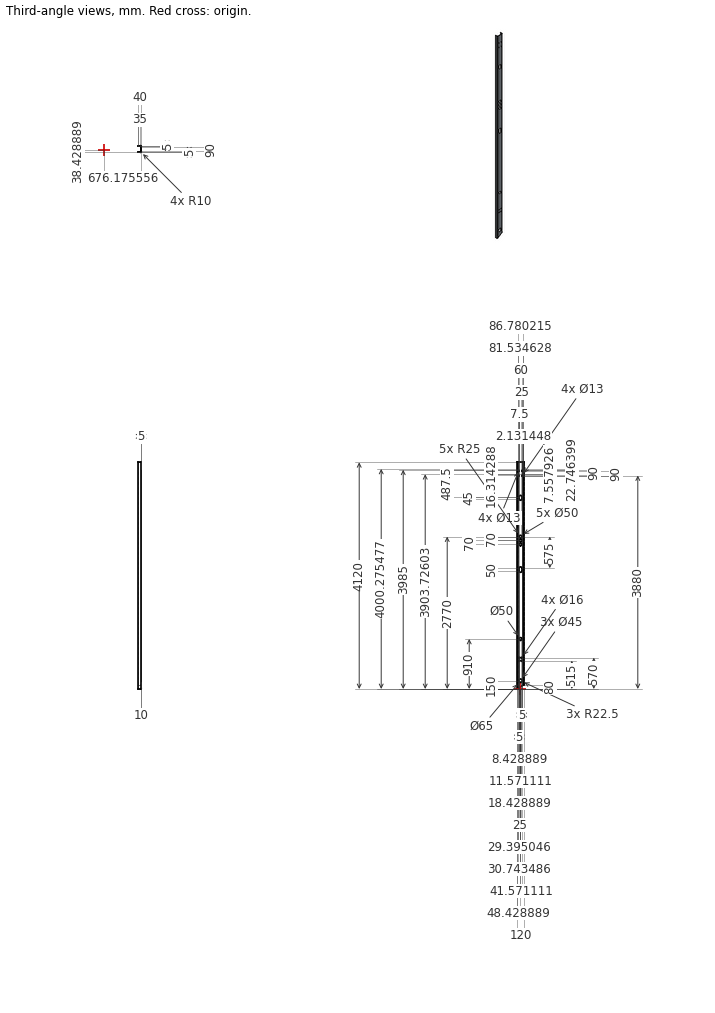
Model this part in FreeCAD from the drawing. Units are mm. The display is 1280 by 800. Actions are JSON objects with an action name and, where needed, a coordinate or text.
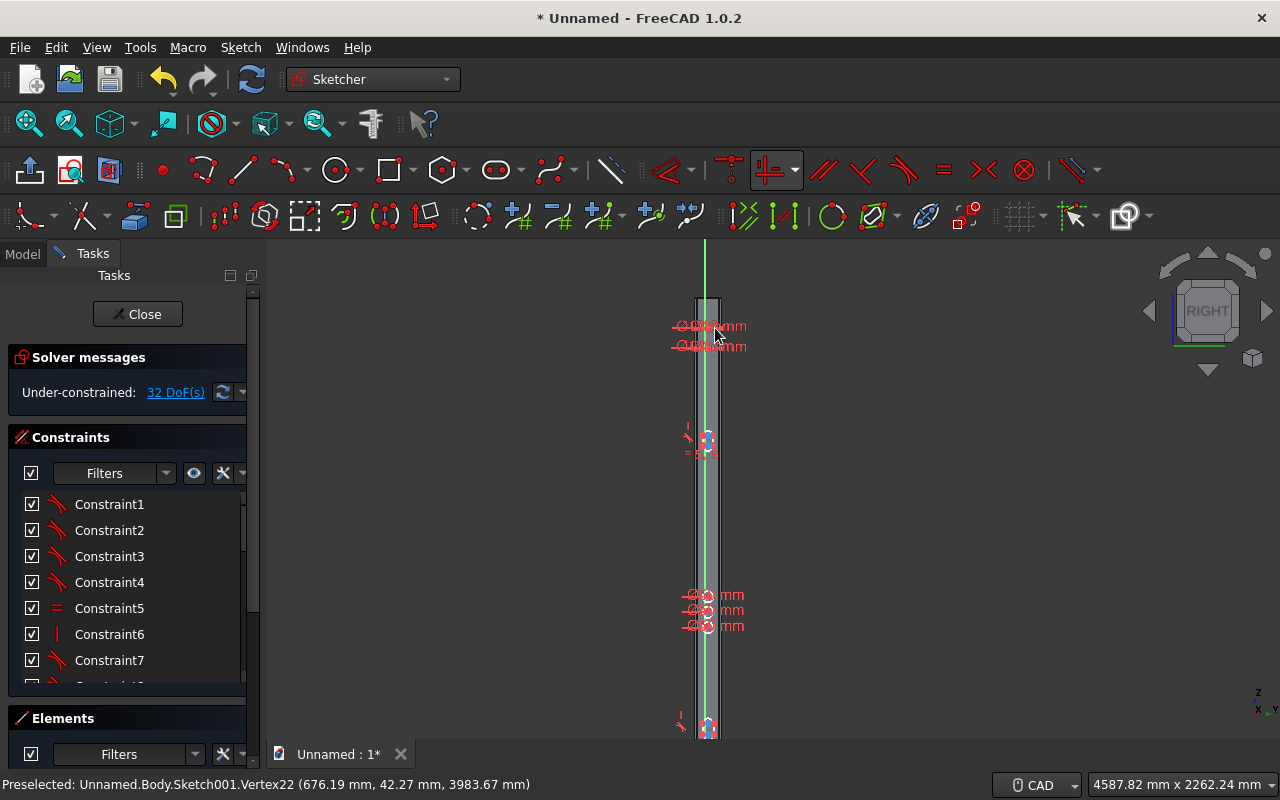
{"action": "key", "text": "h"}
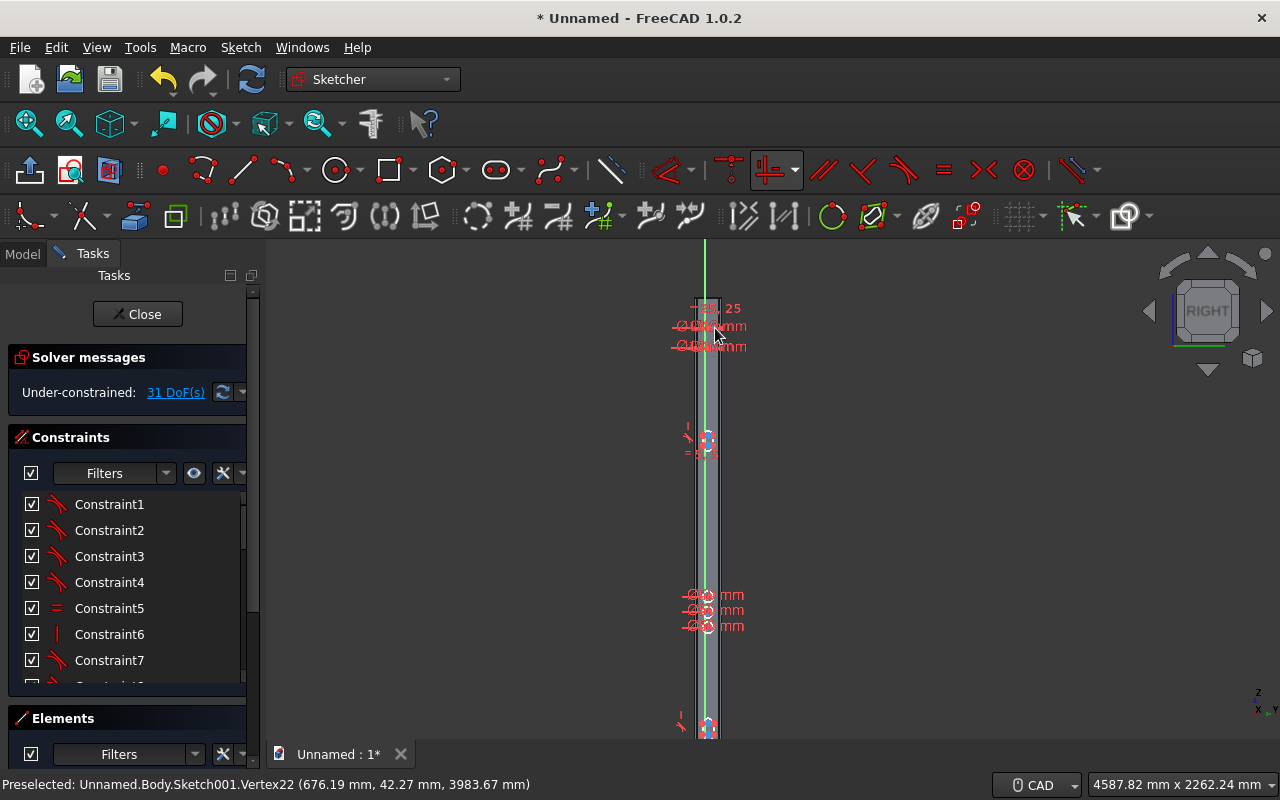
{"action": "left_click", "coordinate": [715, 328]}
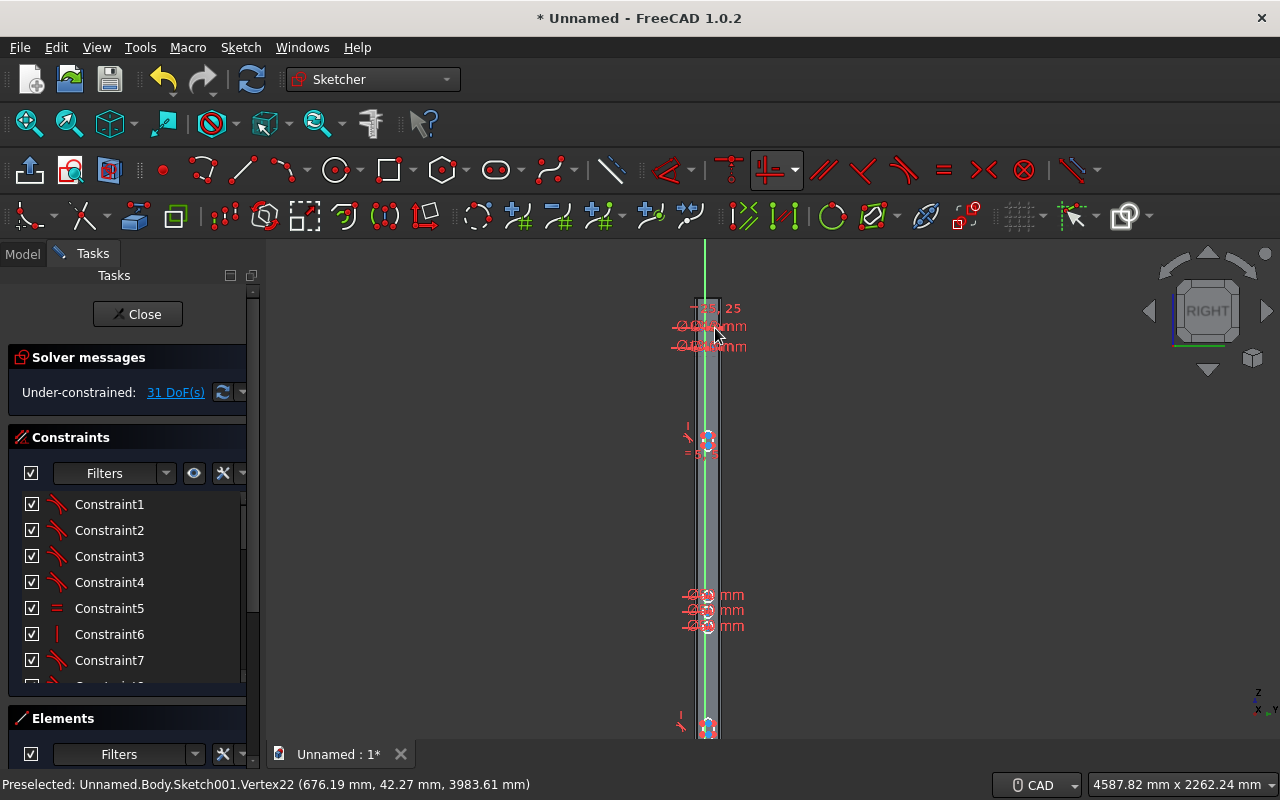
{"action": "left_click", "coordinate": [715, 349]}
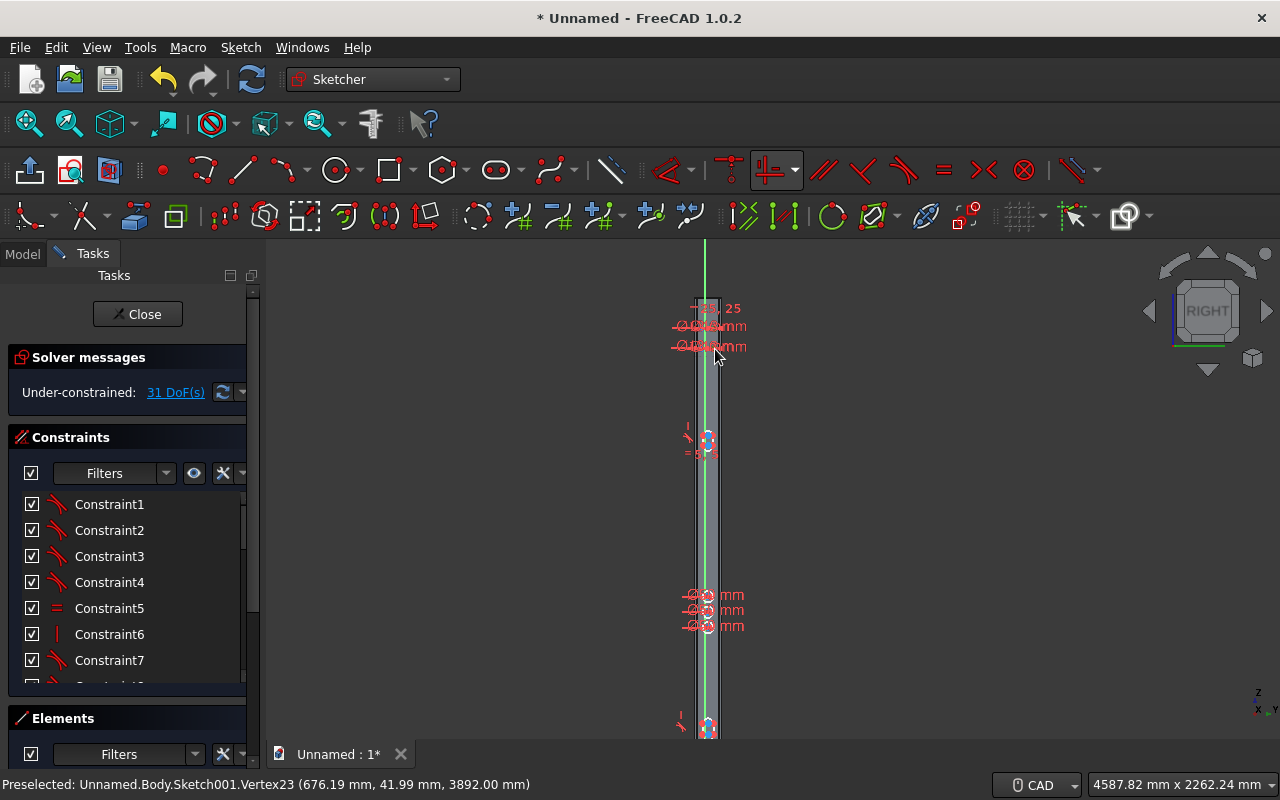
{"action": "left_click", "coordinate": [798, 170]}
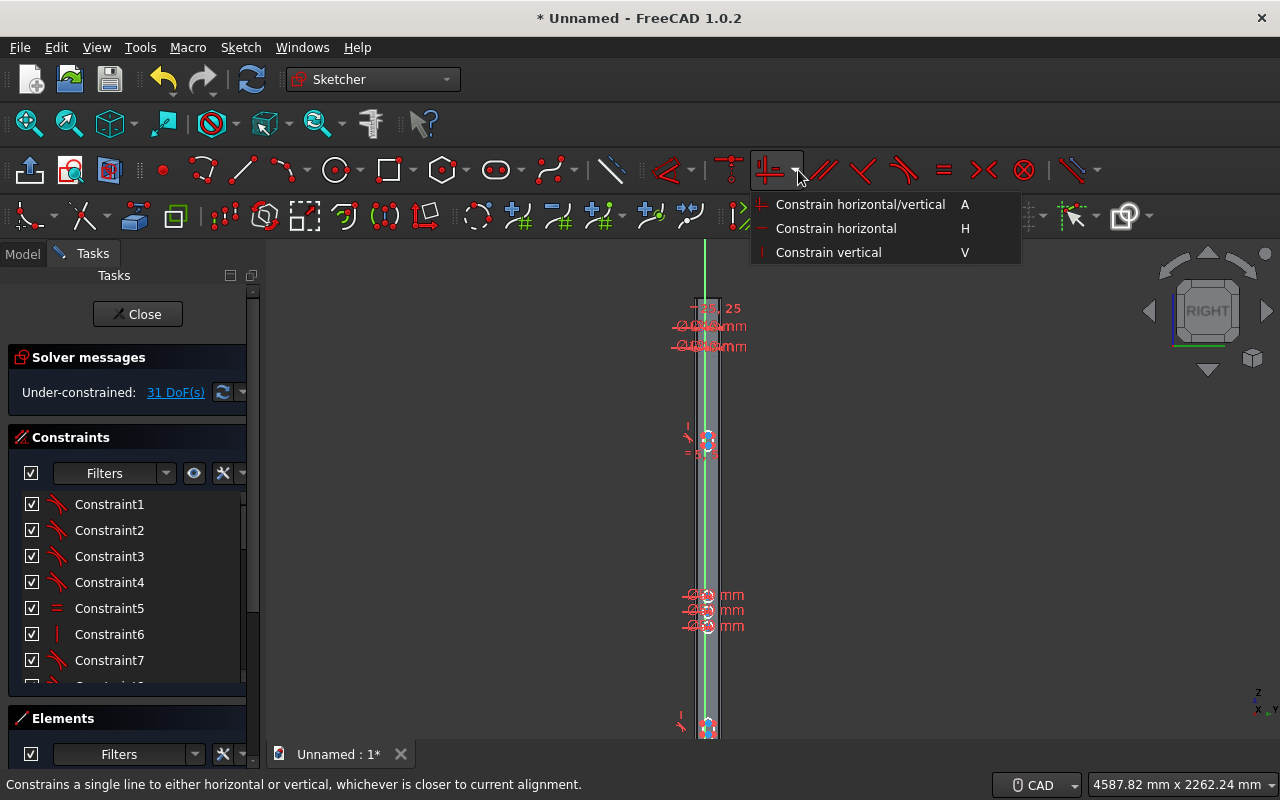
{"action": "left_click", "coordinate": [886, 252]}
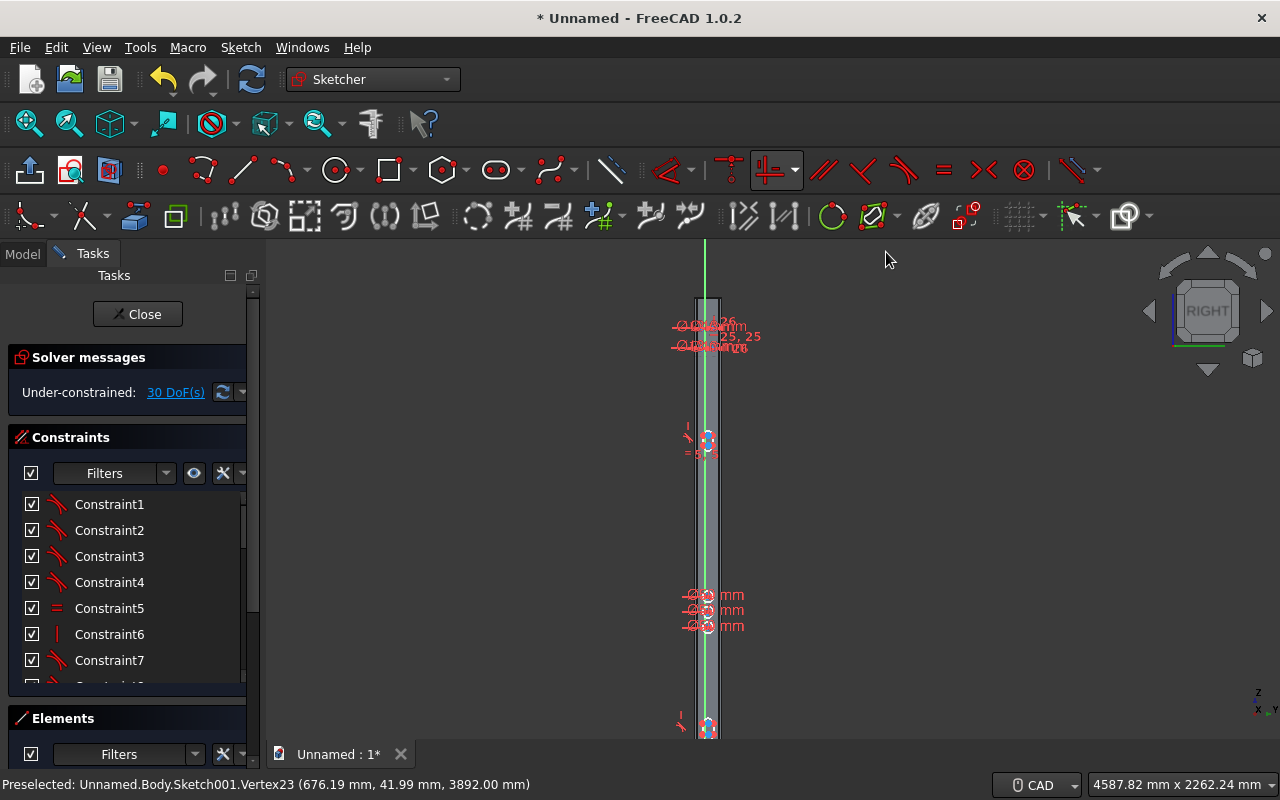
{"action": "left_click", "coordinate": [701, 328]}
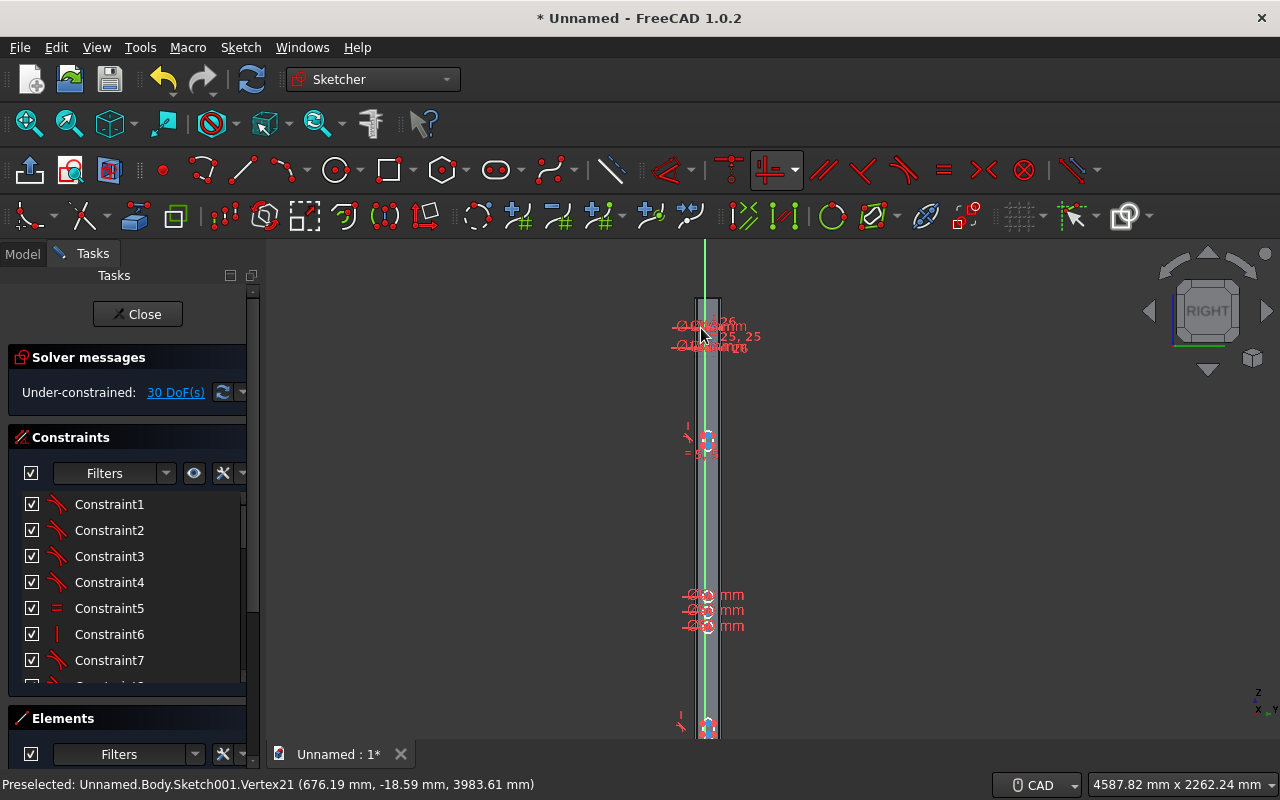
{"action": "left_click", "coordinate": [701, 348]}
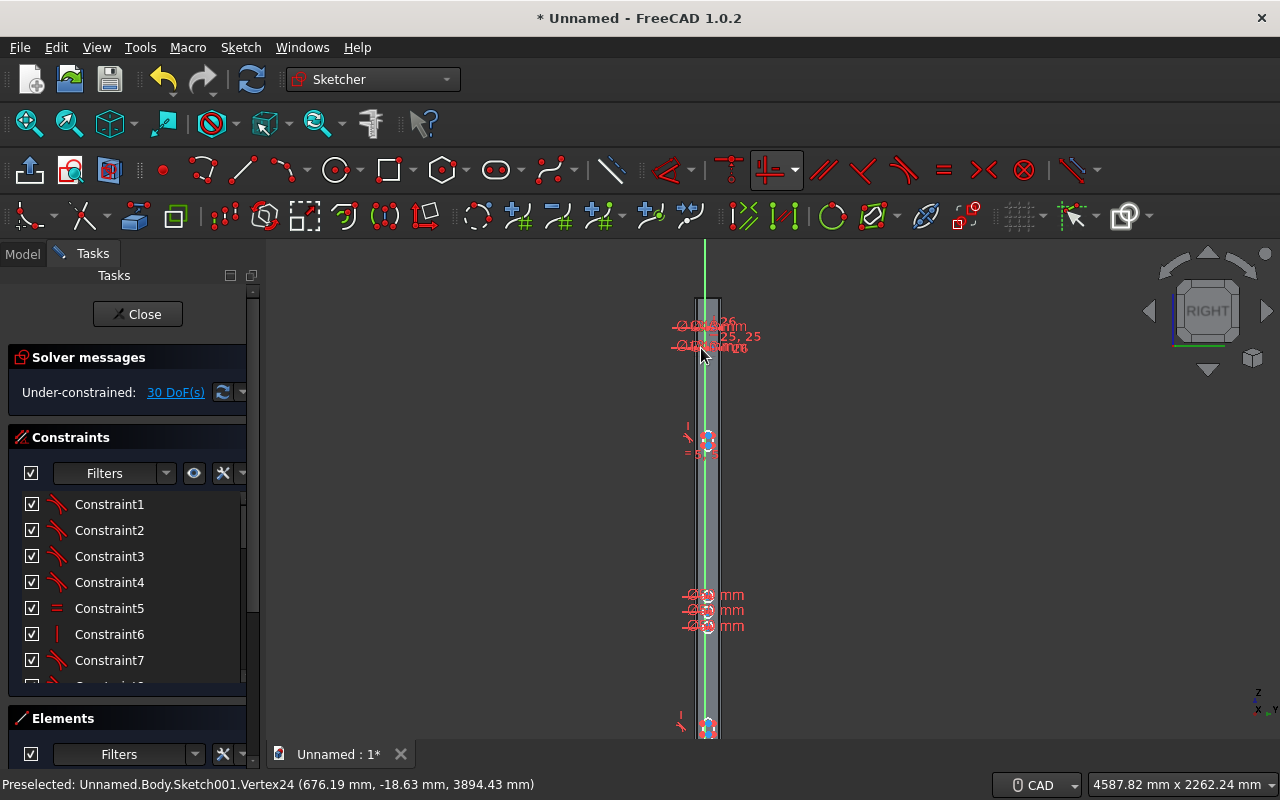
{"action": "key", "text": "v"}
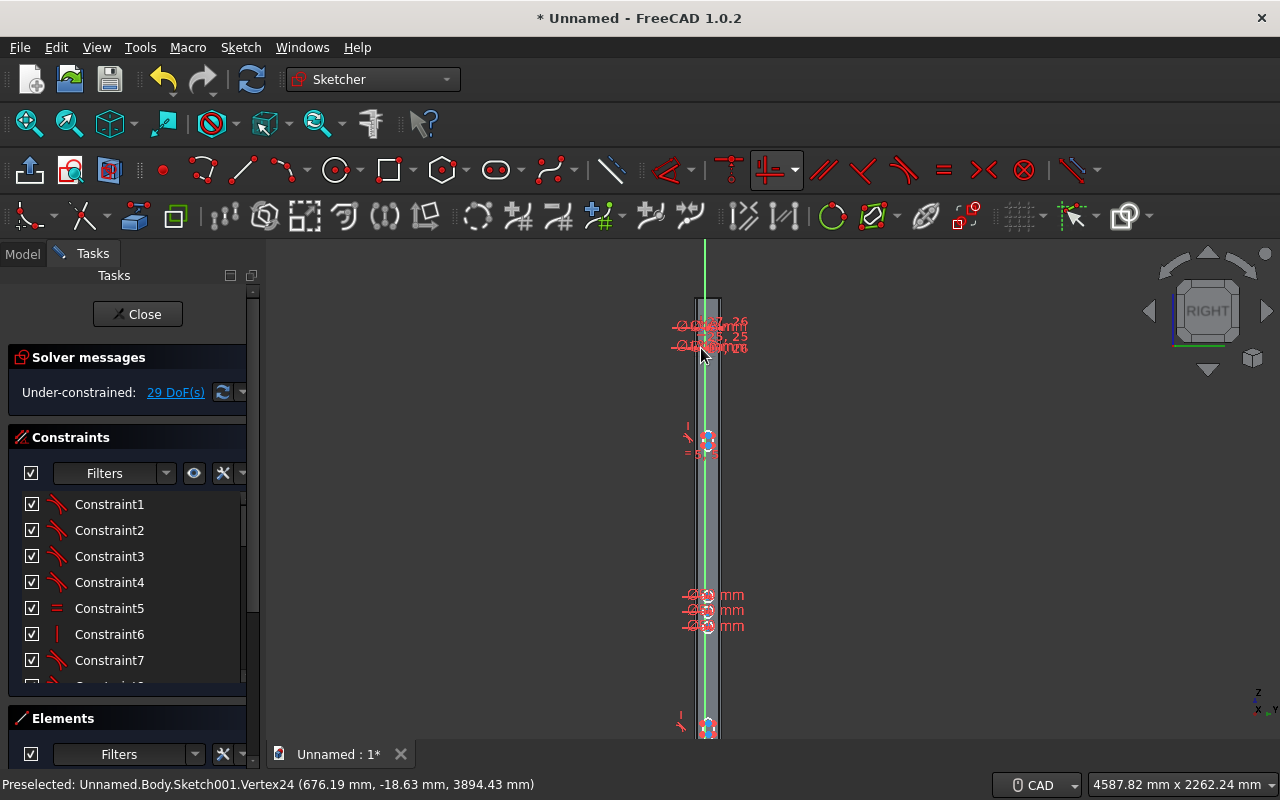
{"action": "scroll", "coordinate": [715, 349], "scroll_direction": "up", "scroll_amount": 4}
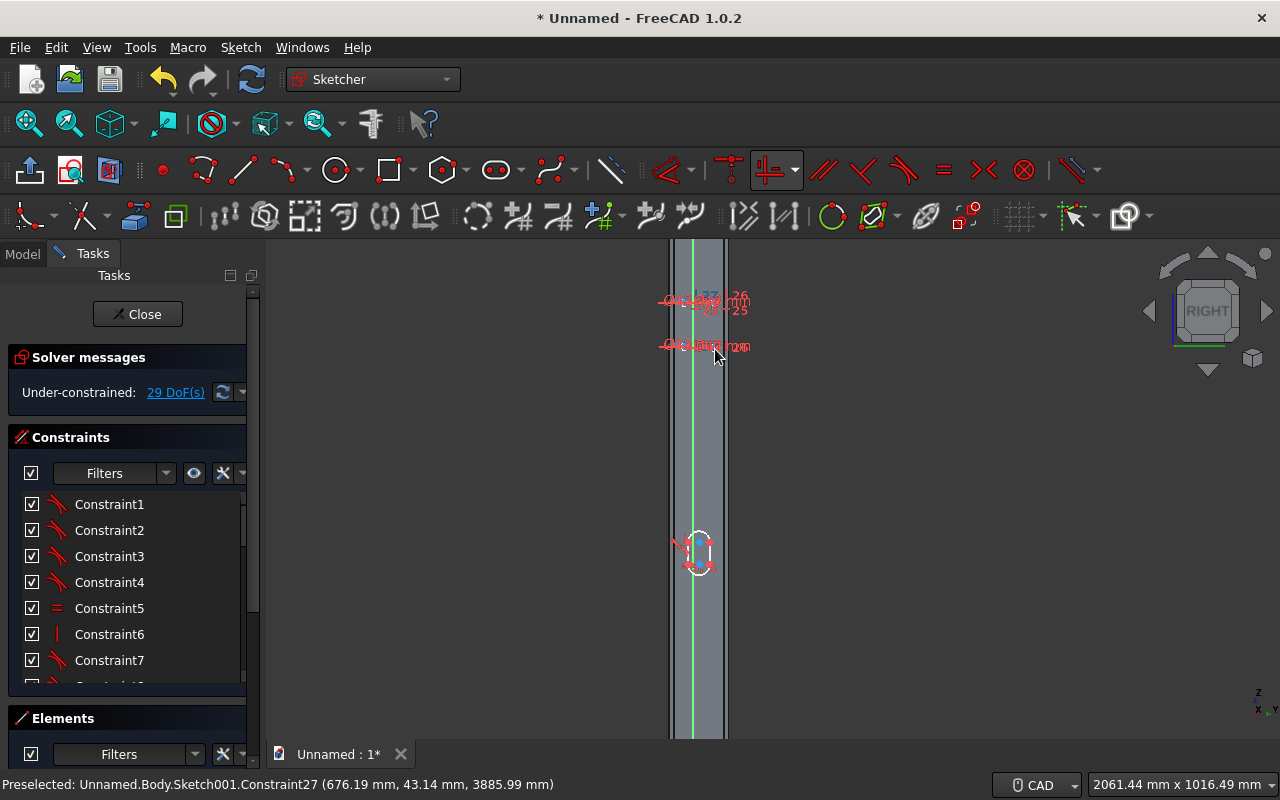
{"action": "scroll", "coordinate": [714, 348], "scroll_direction": "up", "scroll_amount": 4}